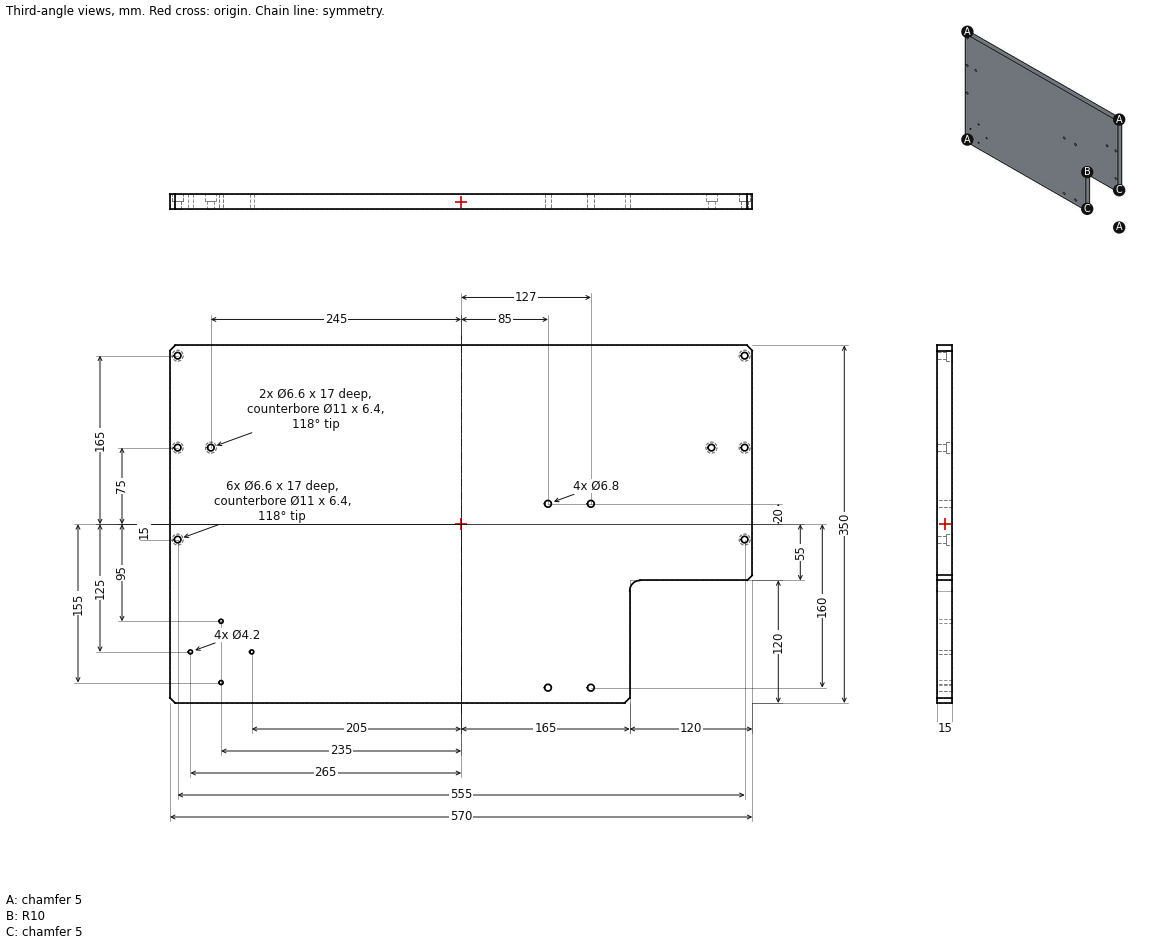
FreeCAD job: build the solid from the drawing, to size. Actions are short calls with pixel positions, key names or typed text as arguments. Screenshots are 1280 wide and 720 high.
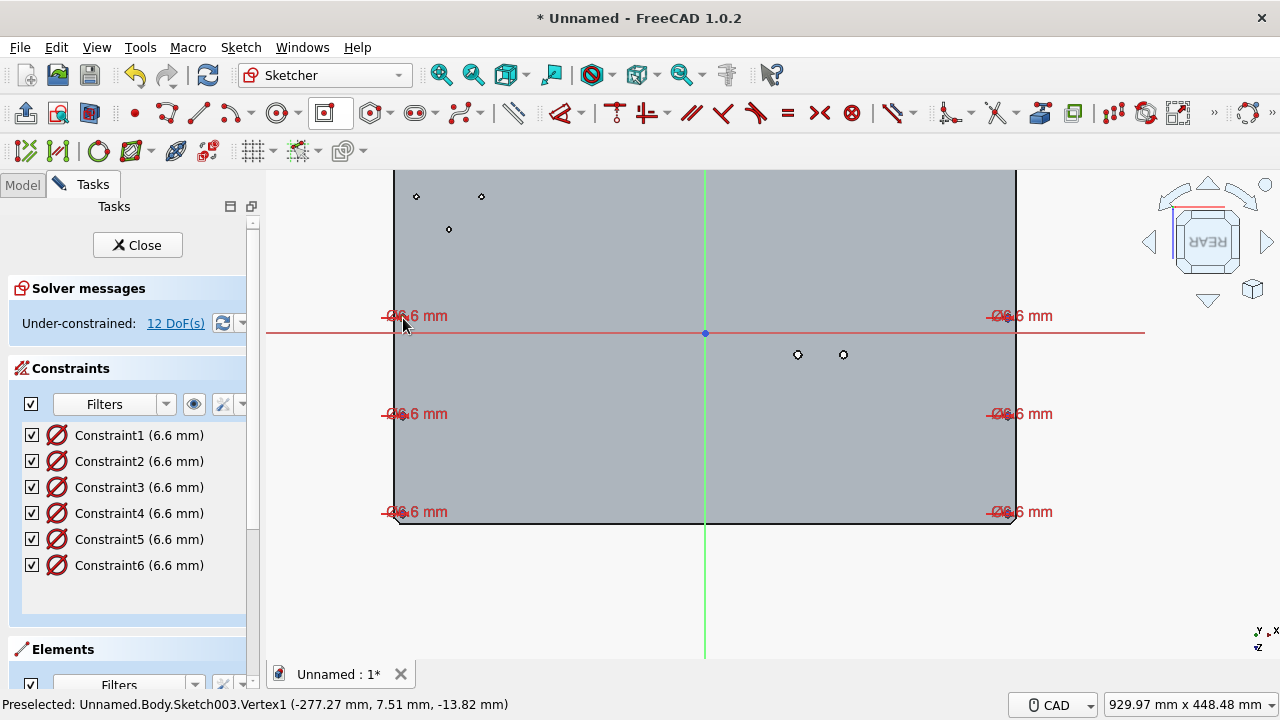
click(1008, 318)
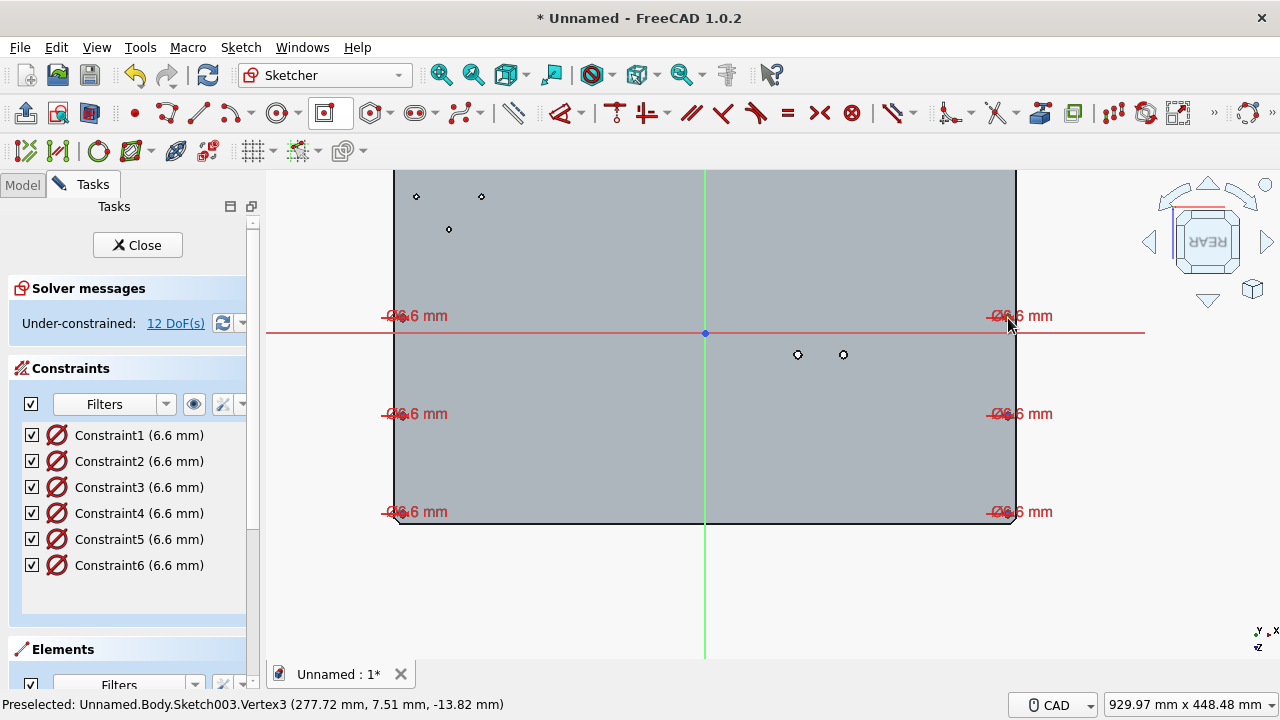
click(705, 600)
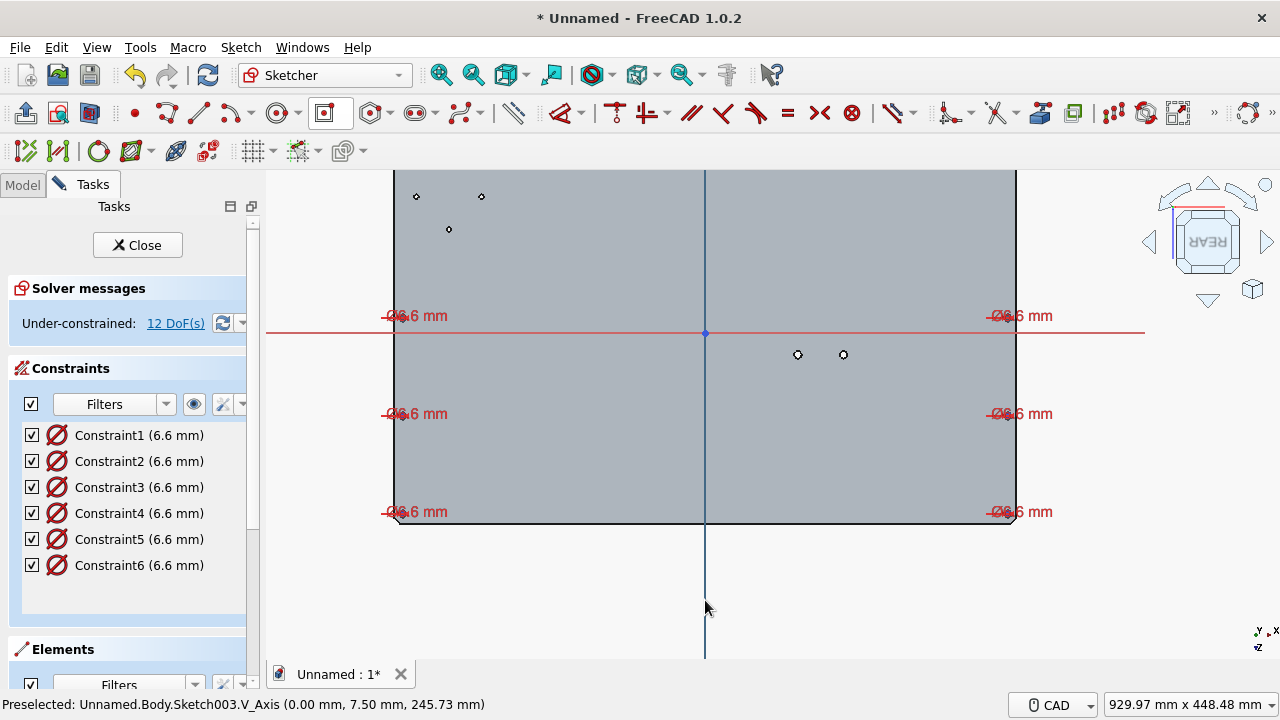
click(820, 114)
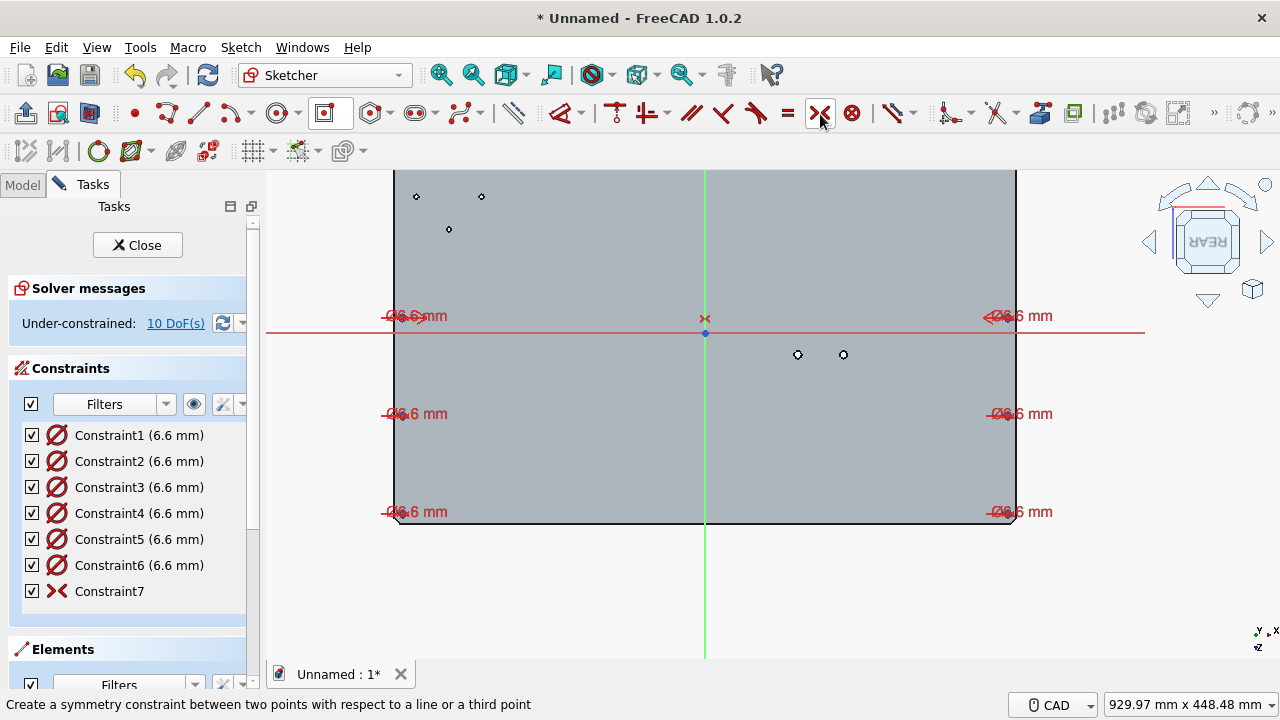
click(403, 514)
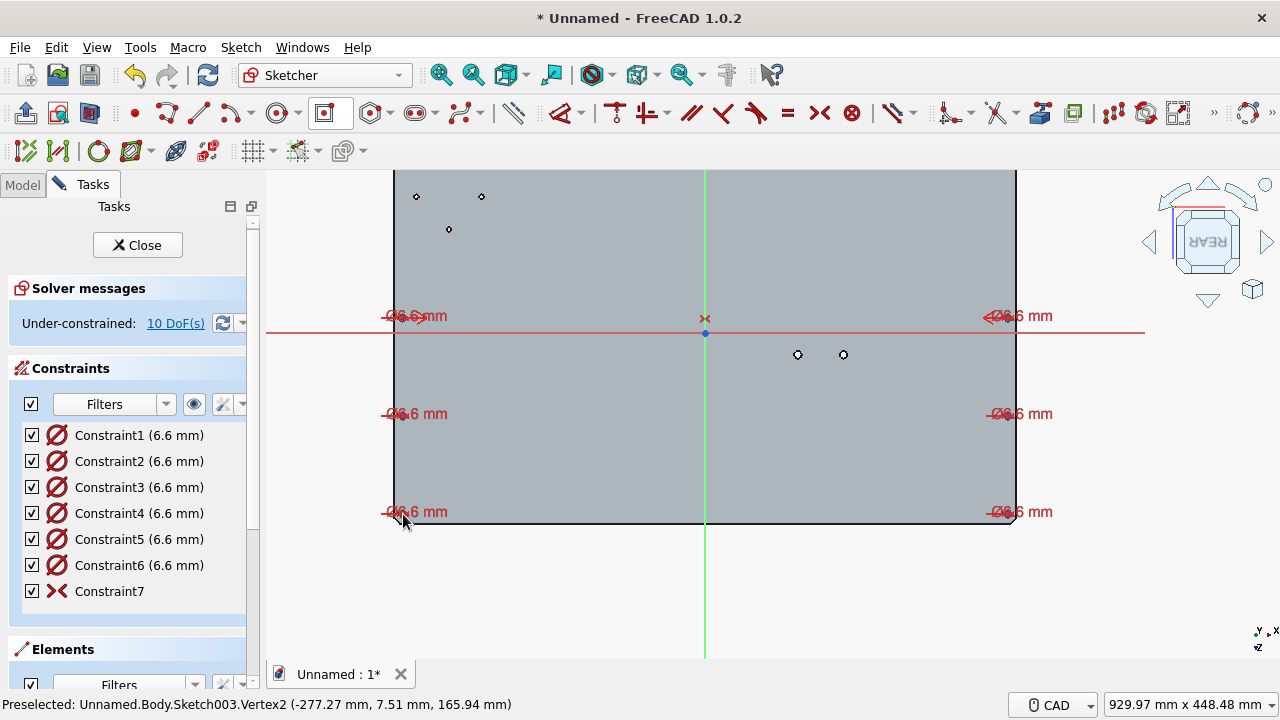
click(1008, 514)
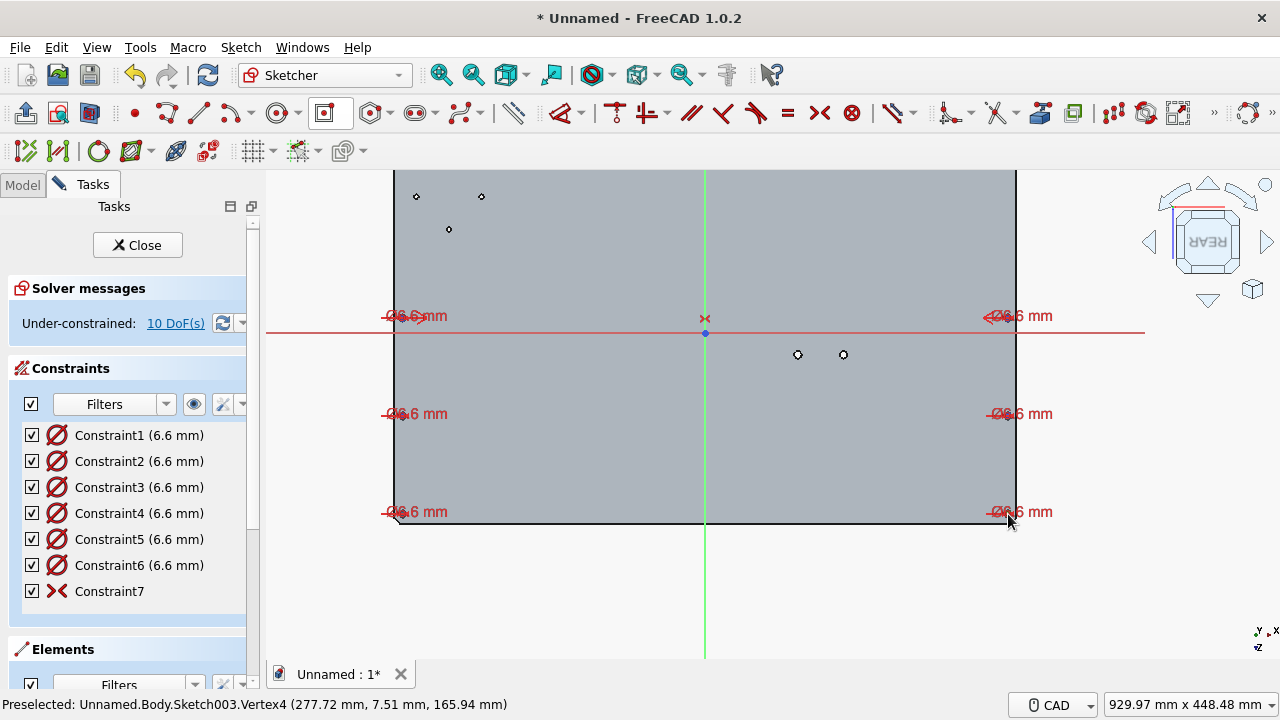
click(705, 600)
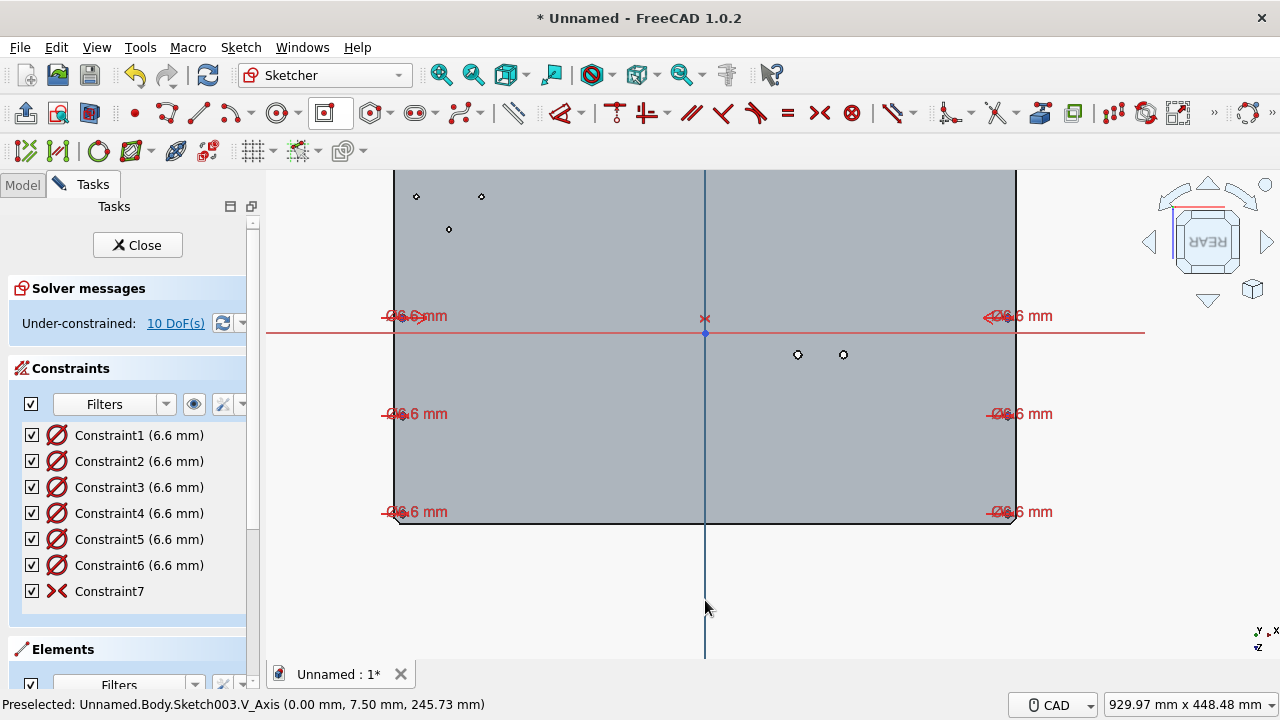
click(820, 114)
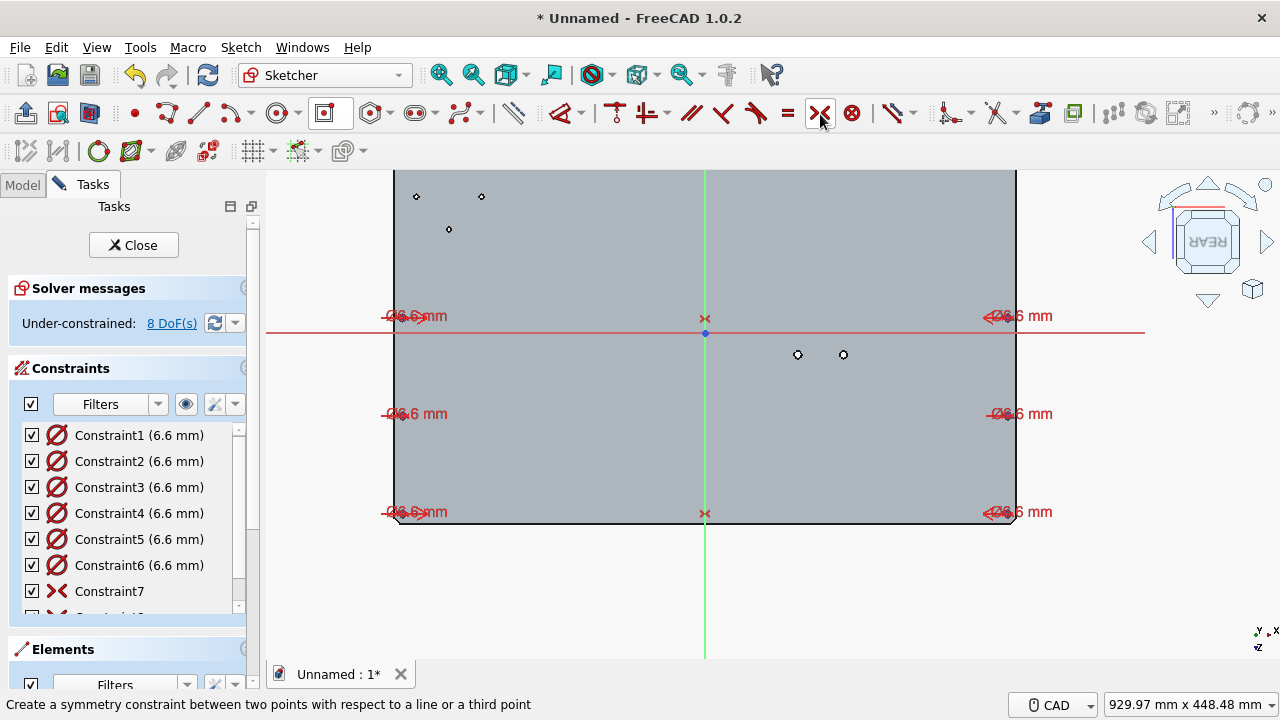
click(403, 416)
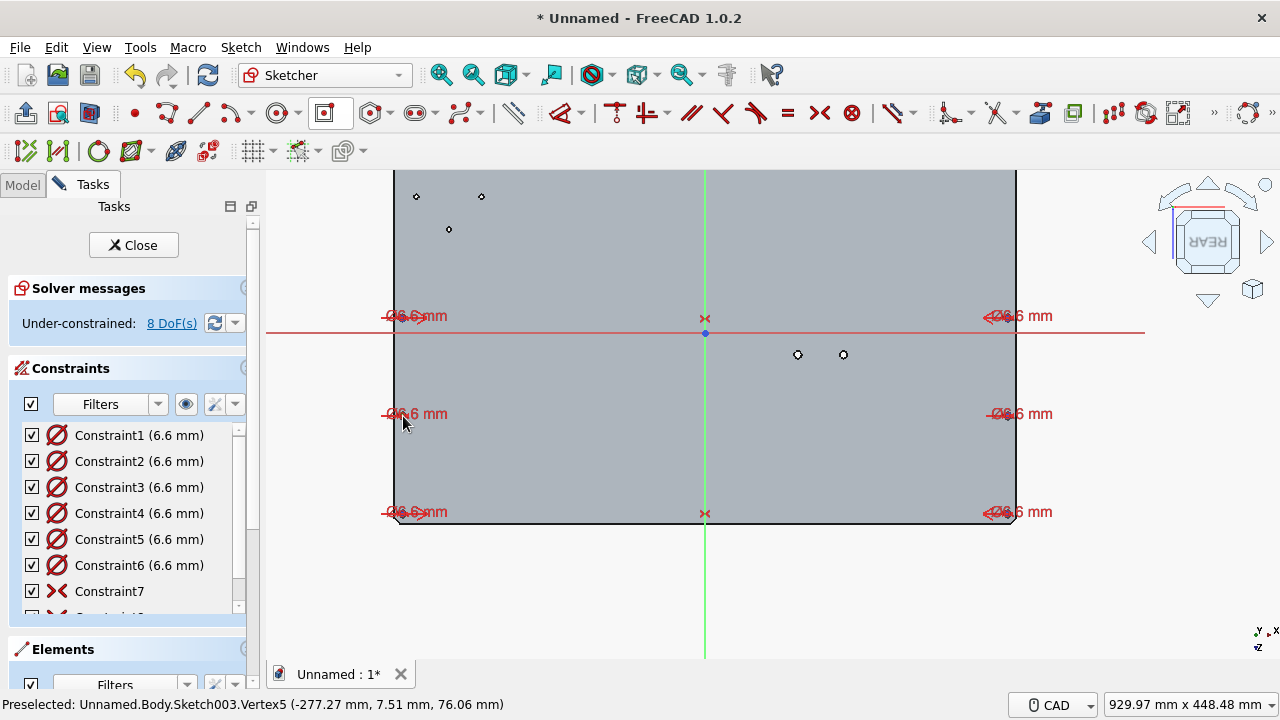
click(1008, 416)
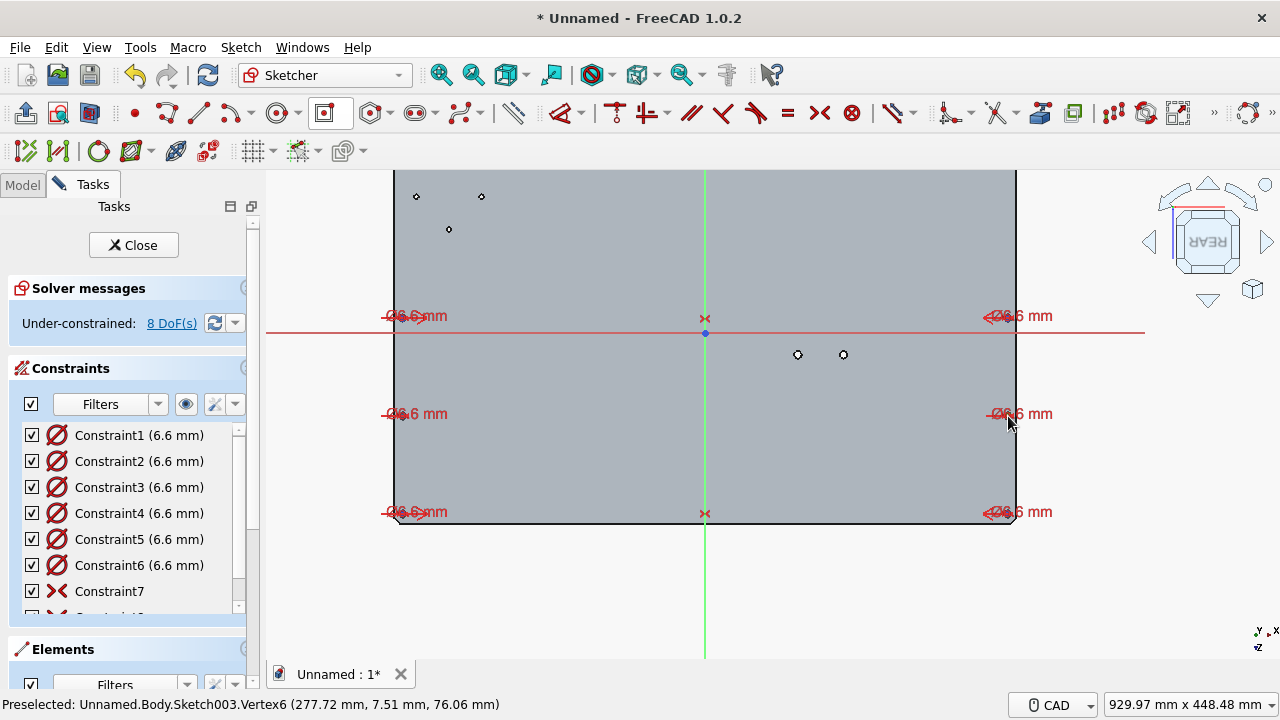
click(705, 600)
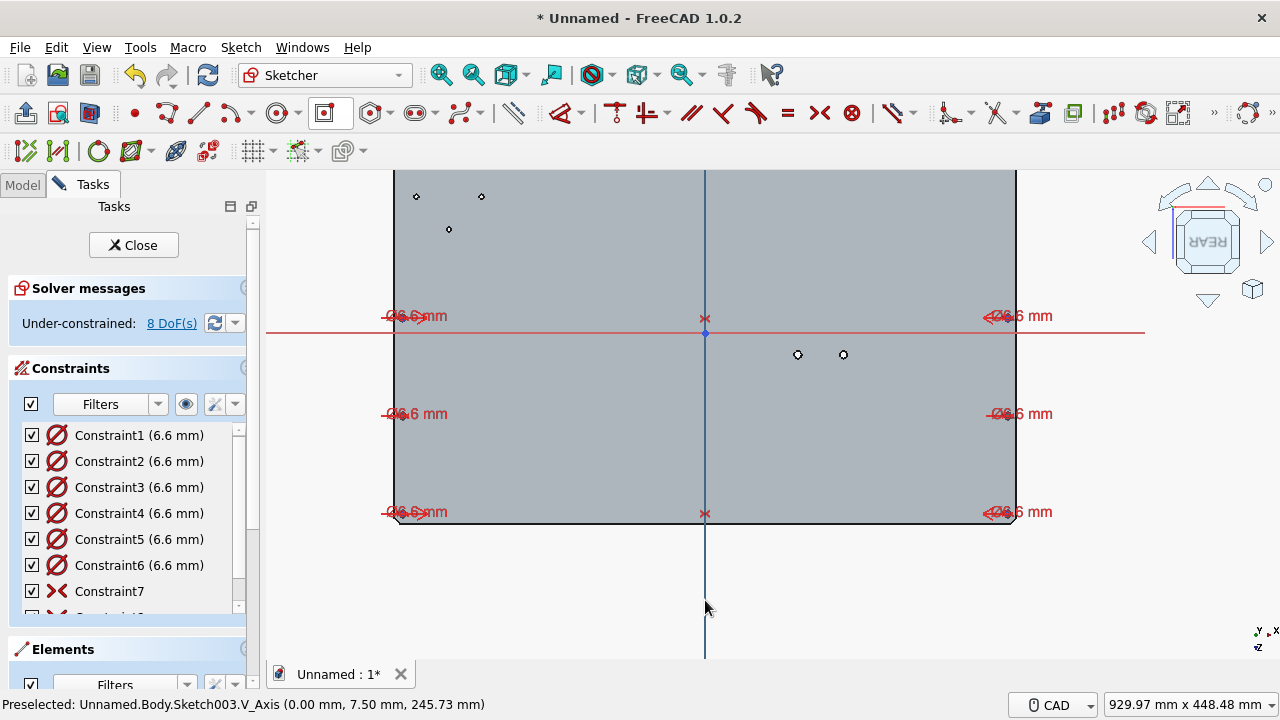
click(820, 114)